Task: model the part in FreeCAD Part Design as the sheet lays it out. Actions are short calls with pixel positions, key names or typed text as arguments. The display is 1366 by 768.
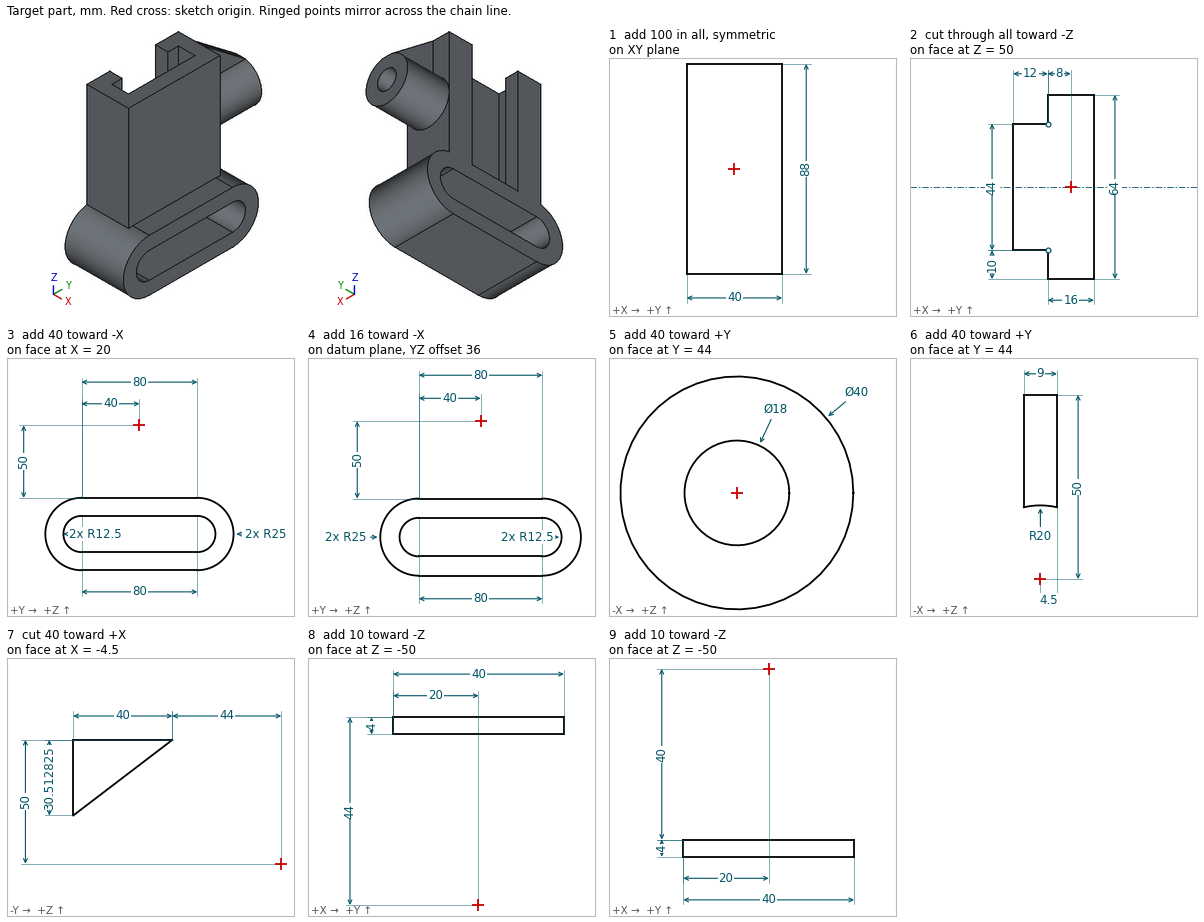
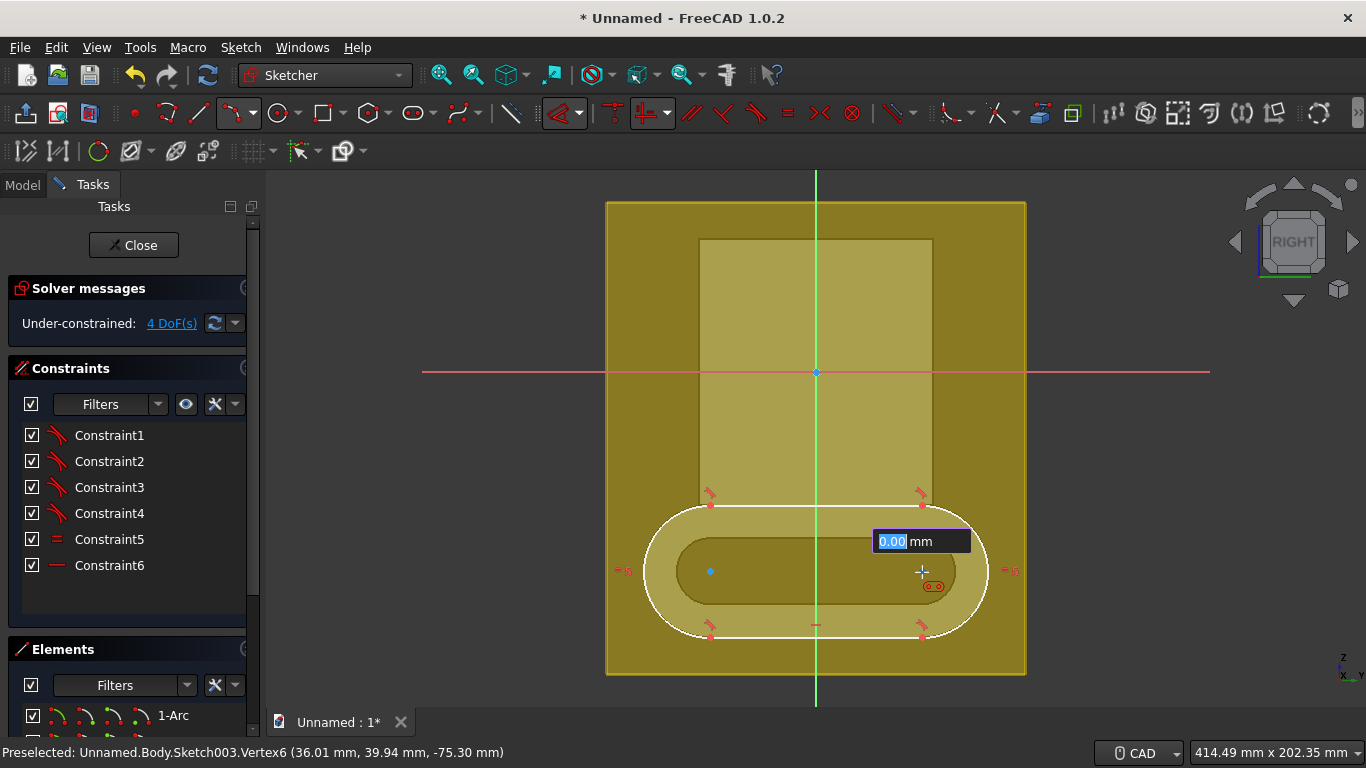
click(784, 538)
key(Escape)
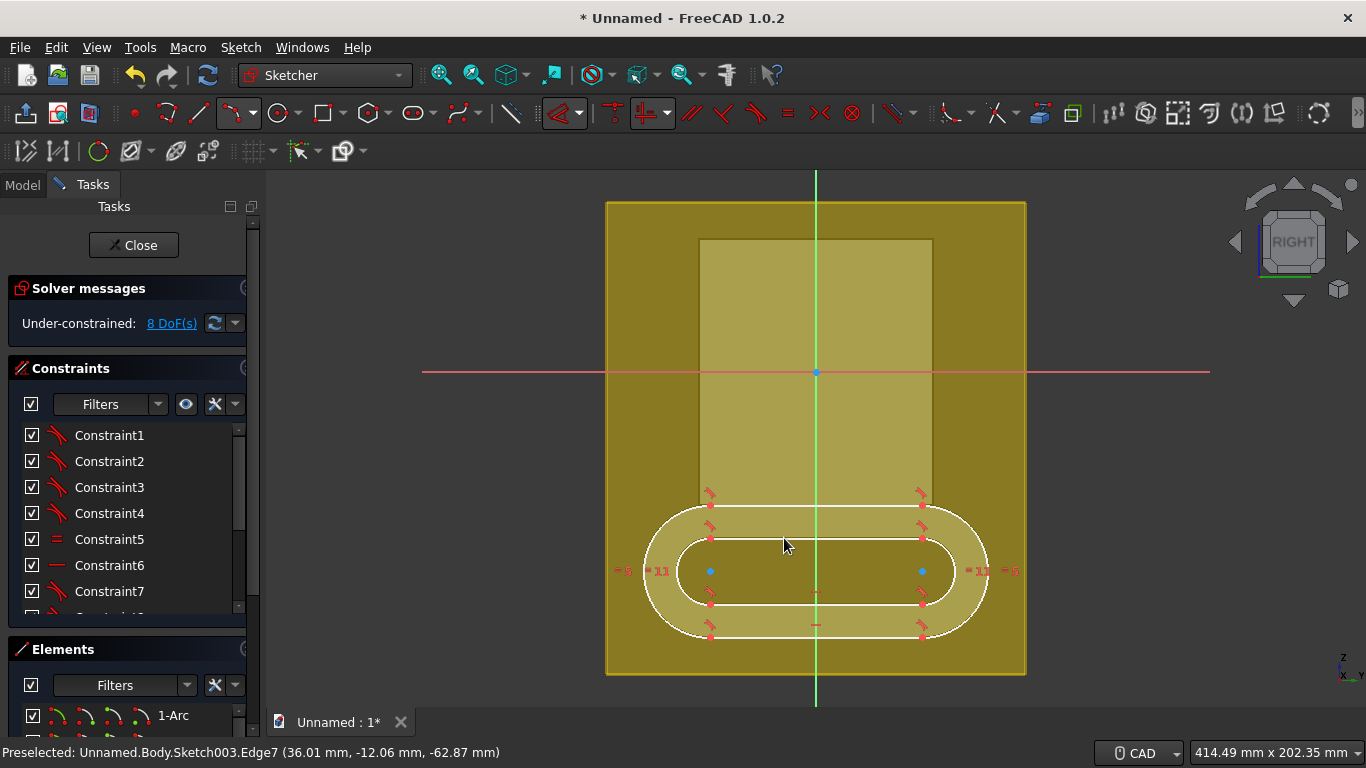
click(657, 533)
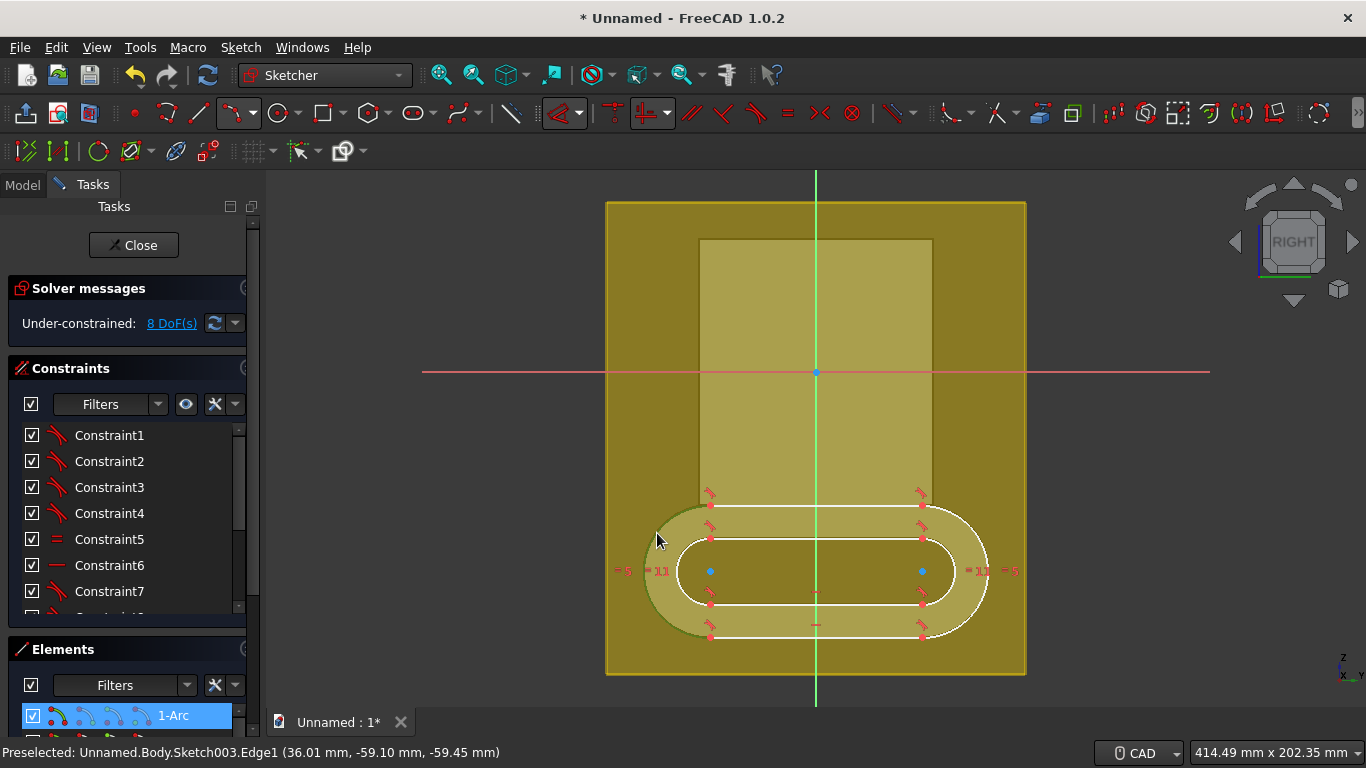
click(683, 553)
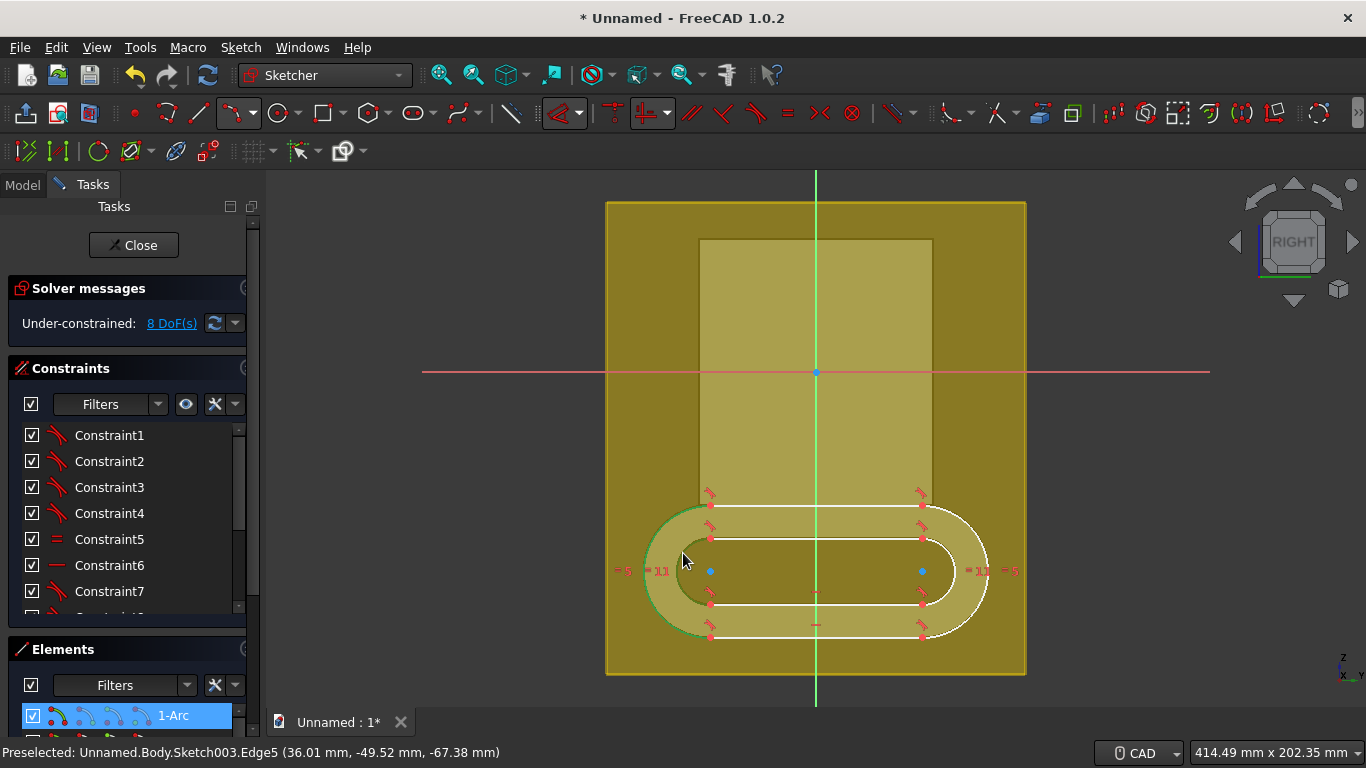
key(c)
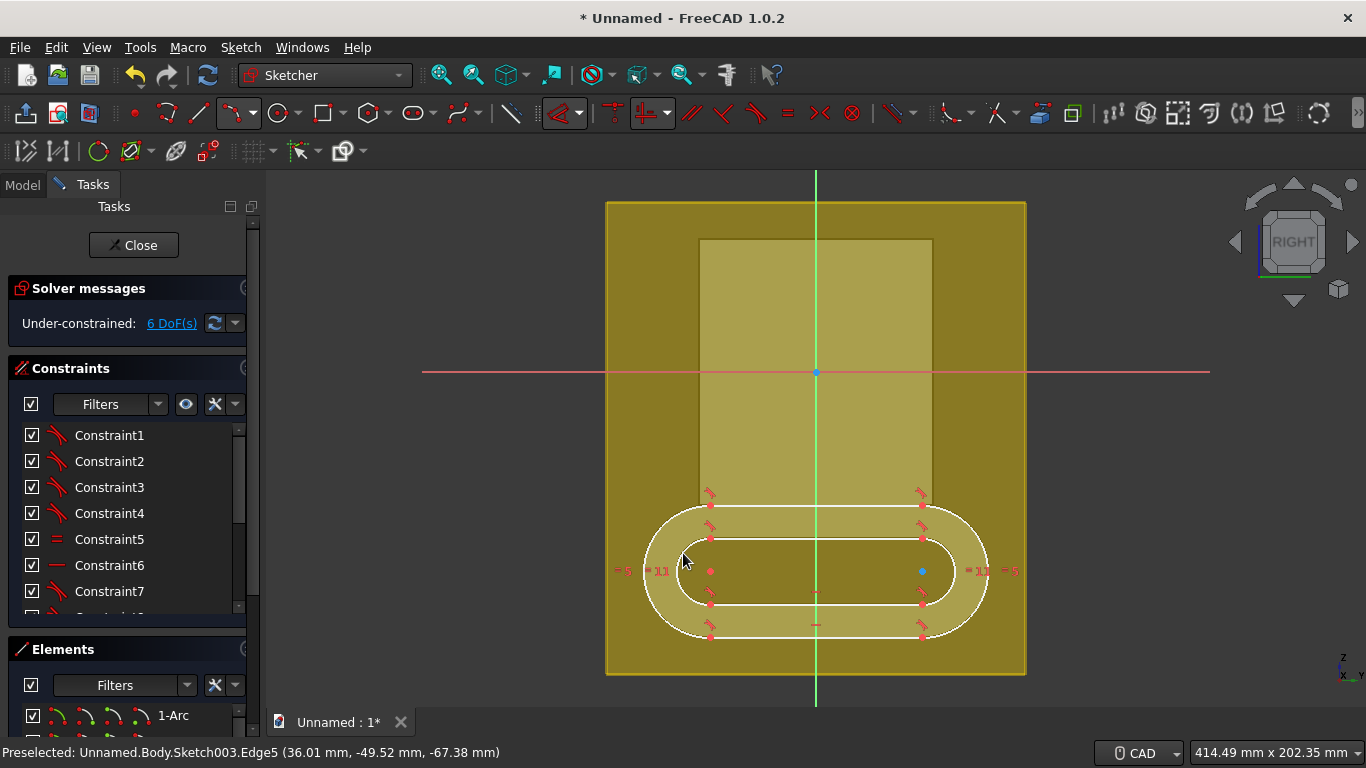
click(657, 533)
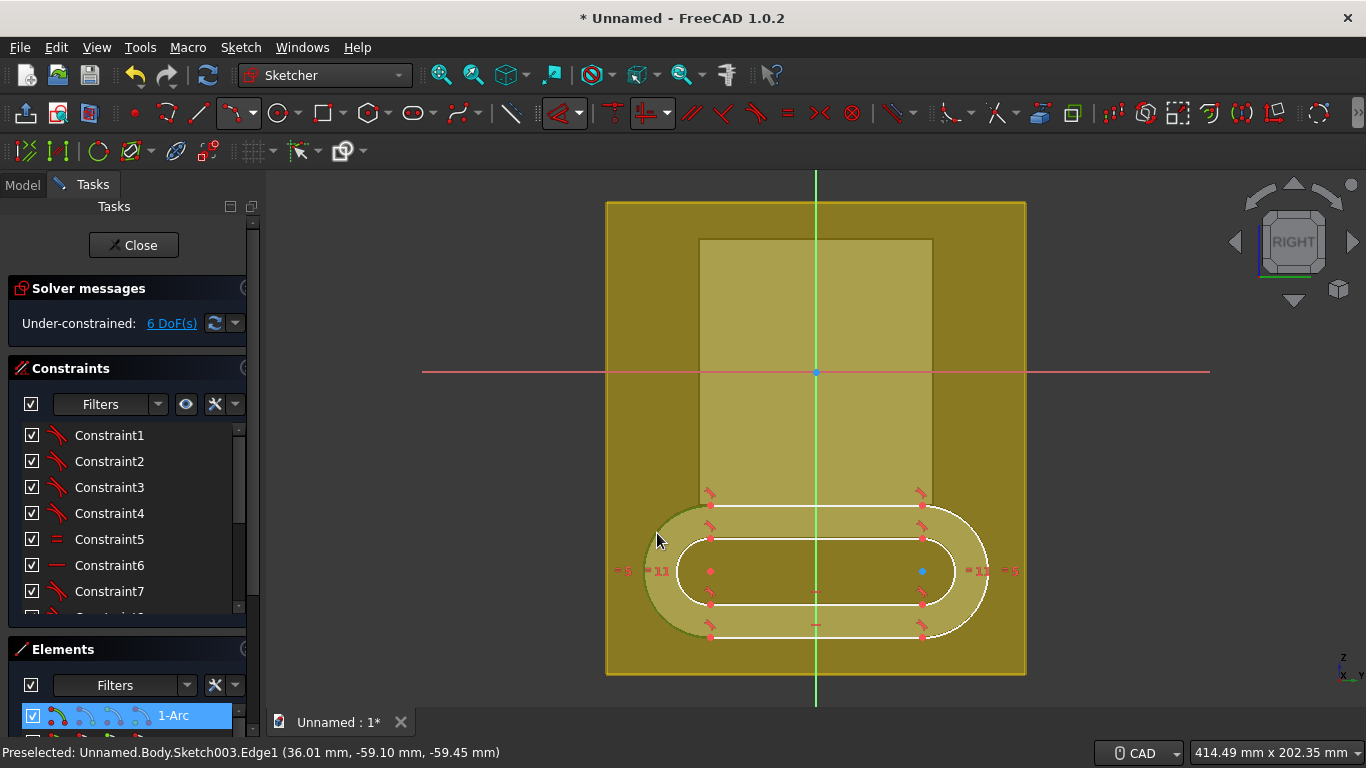
key(k)
key(r)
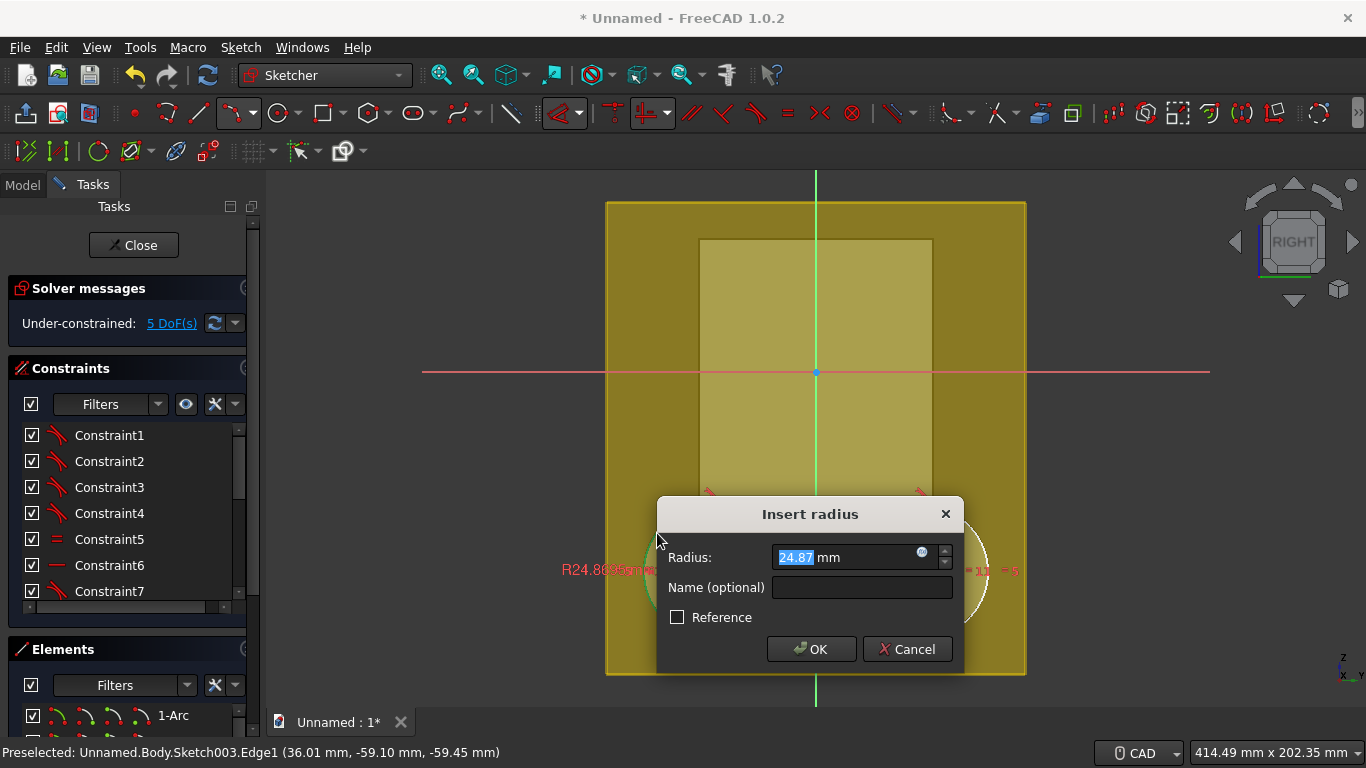
text(25)
key(Return)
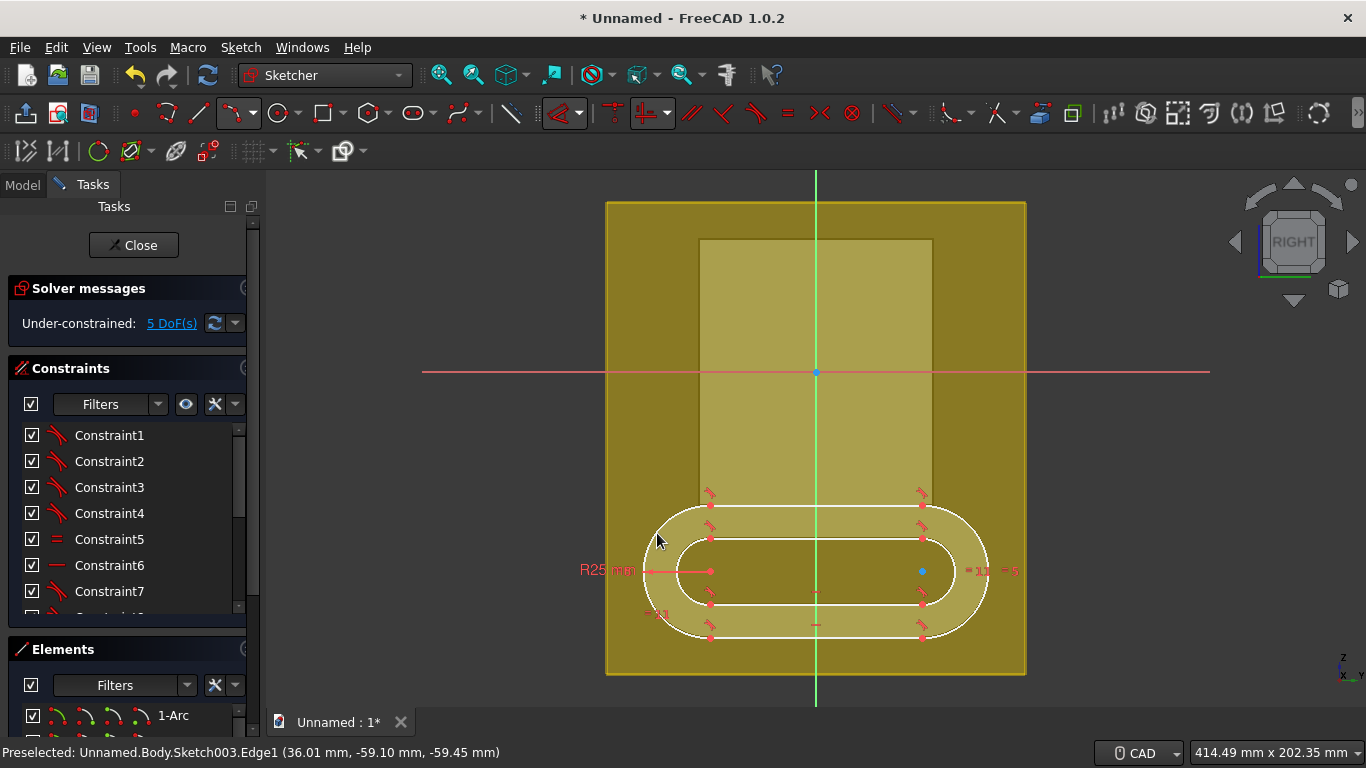
click(683, 553)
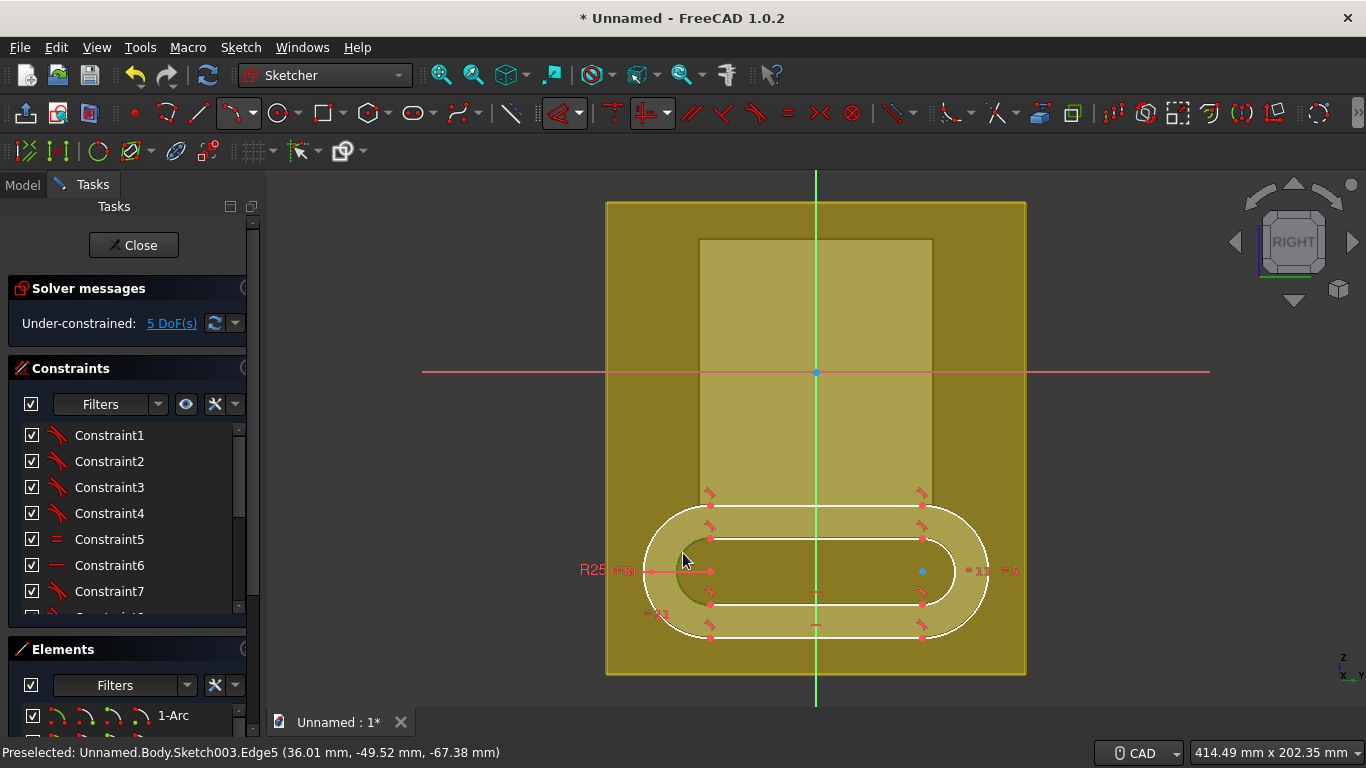
key(k)
key(r)